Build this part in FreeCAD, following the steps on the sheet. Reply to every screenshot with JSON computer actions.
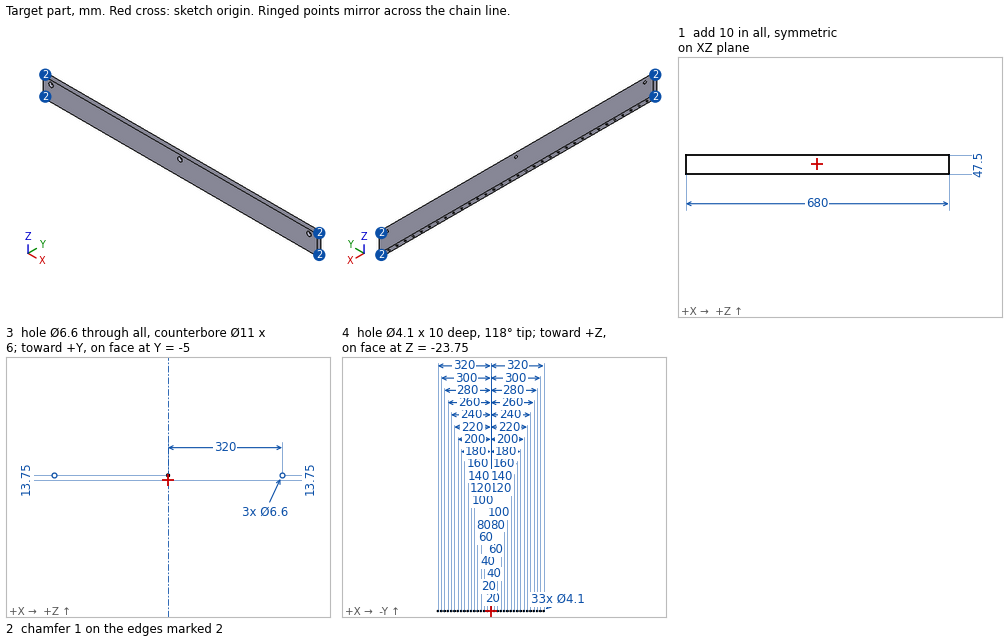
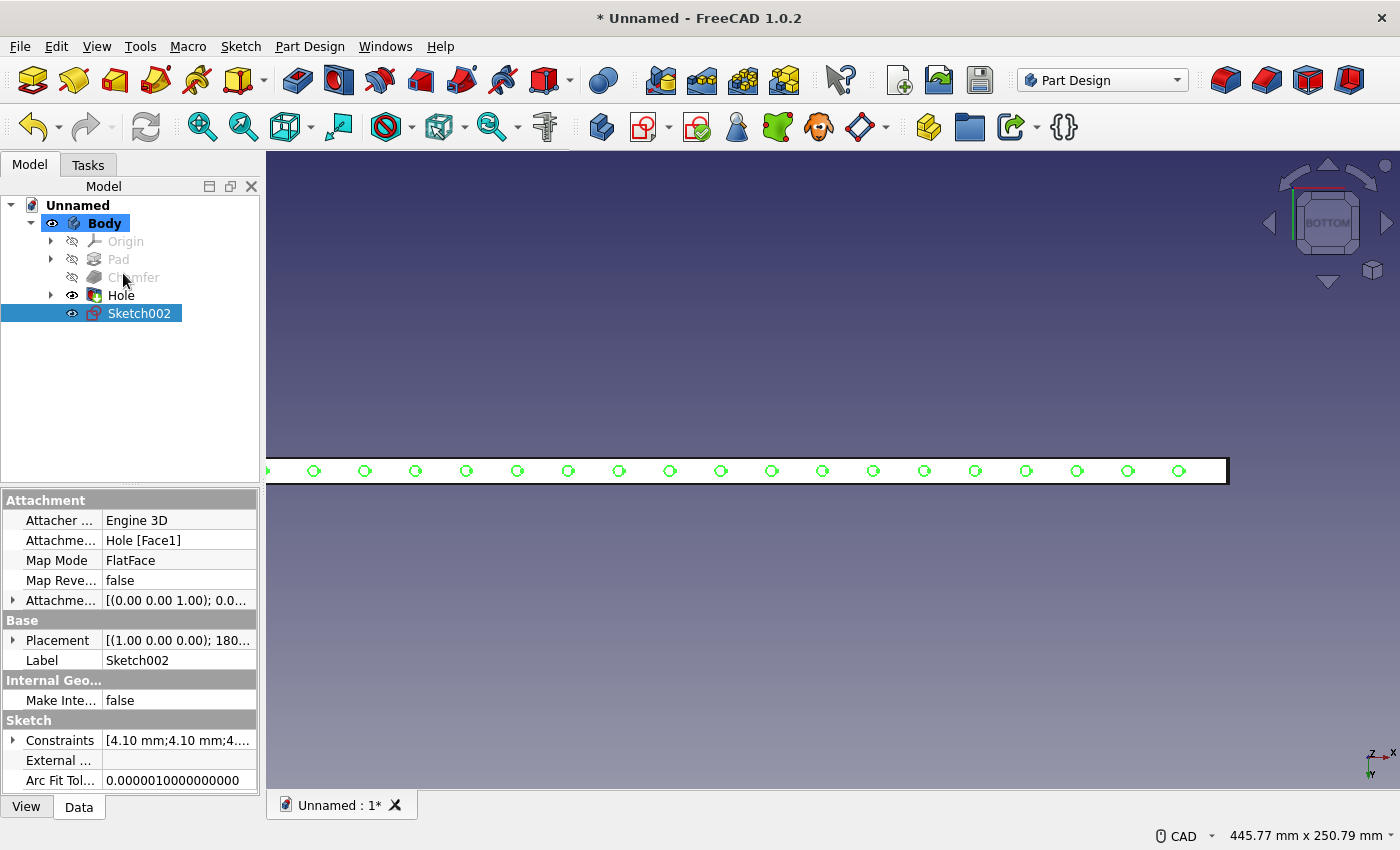
{"action": "left_click", "coordinate": [339, 80]}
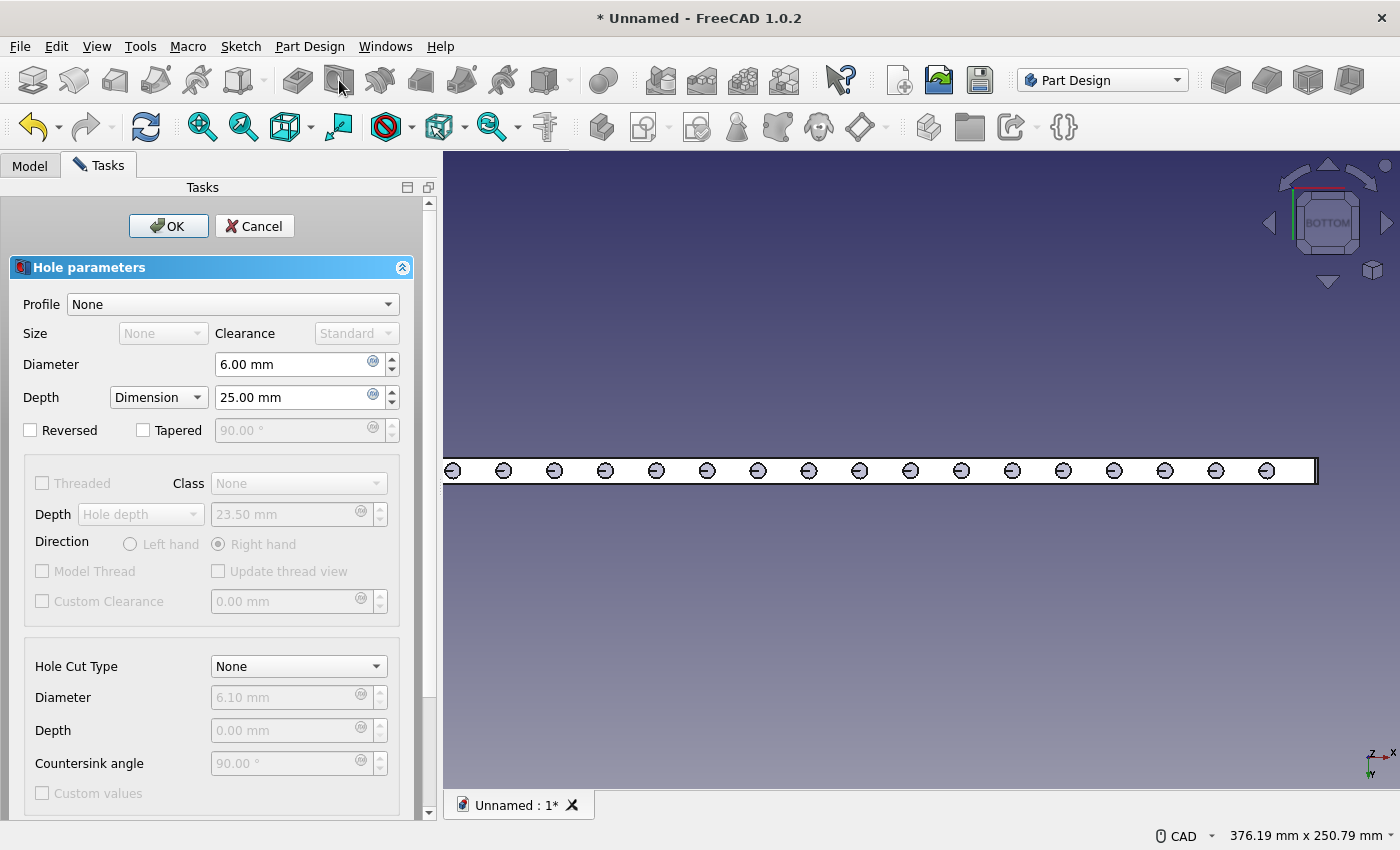
{"action": "triple_click", "coordinate": [300, 364]}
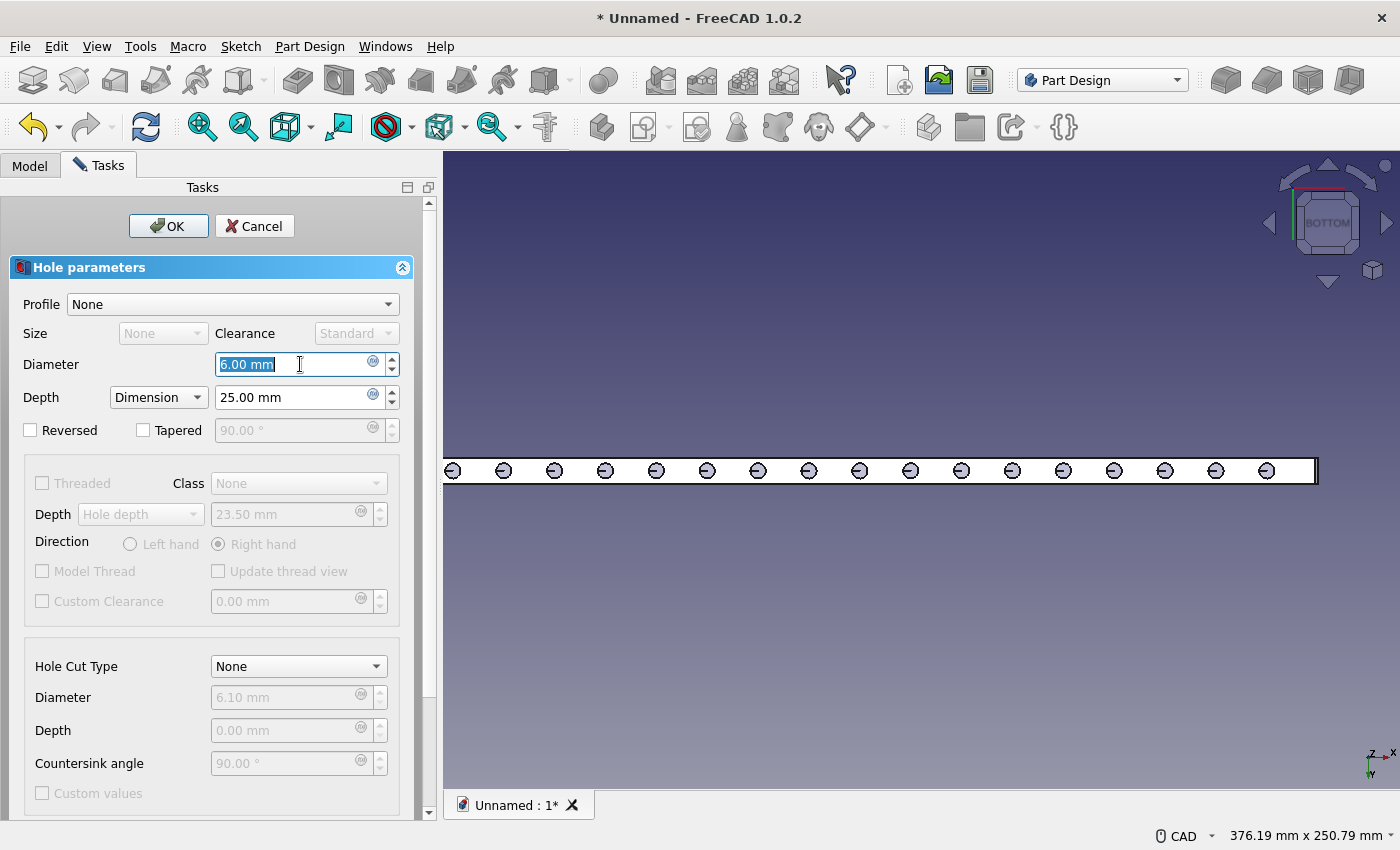
{"action": "type", "text": "4.1"}
{"action": "key", "text": "Tab"}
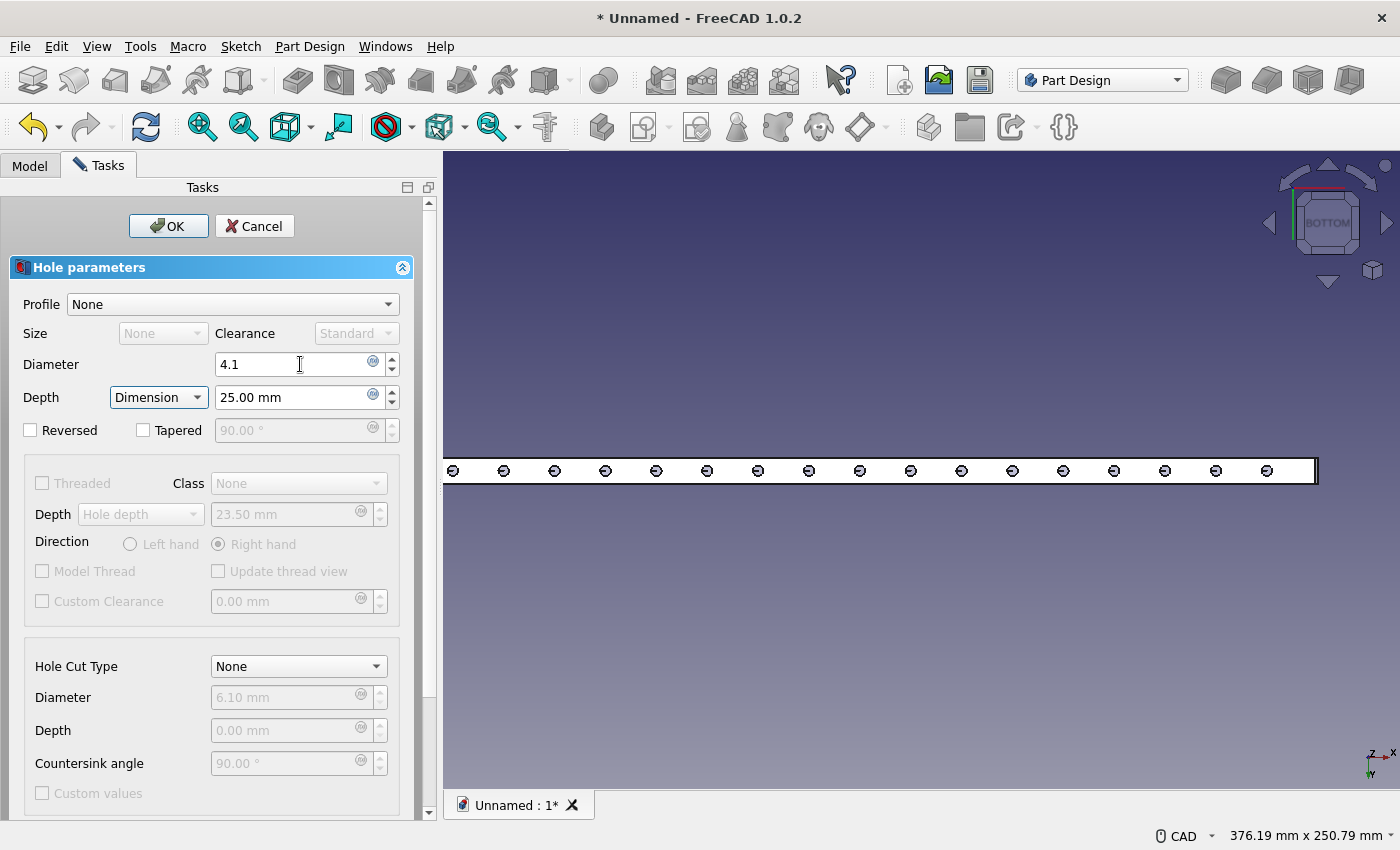
{"action": "triple_click", "coordinate": [300, 398]}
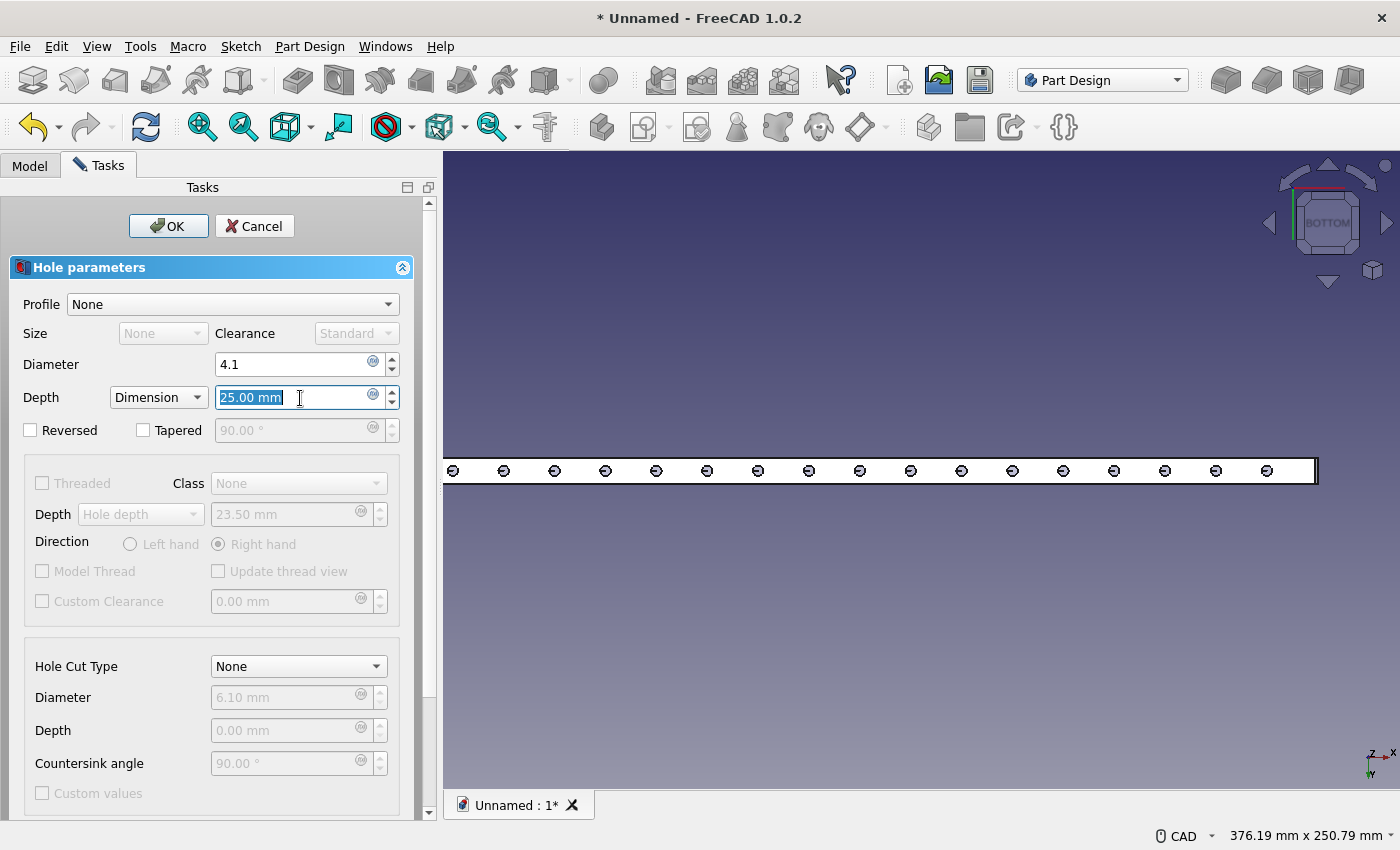
{"action": "type", "text": "10"}
{"action": "key", "text": "Tab"}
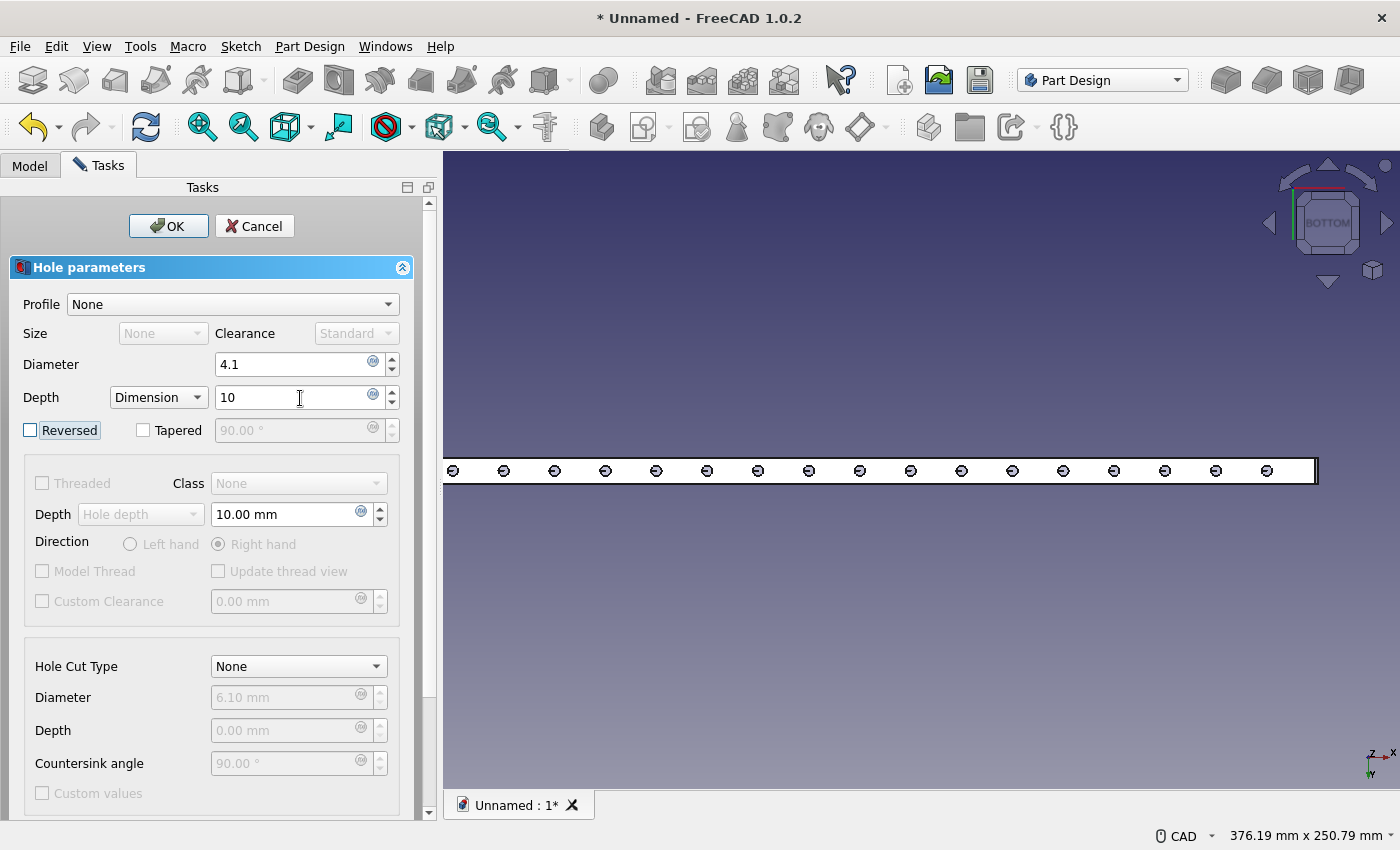
{"action": "left_click", "coordinate": [169, 226]}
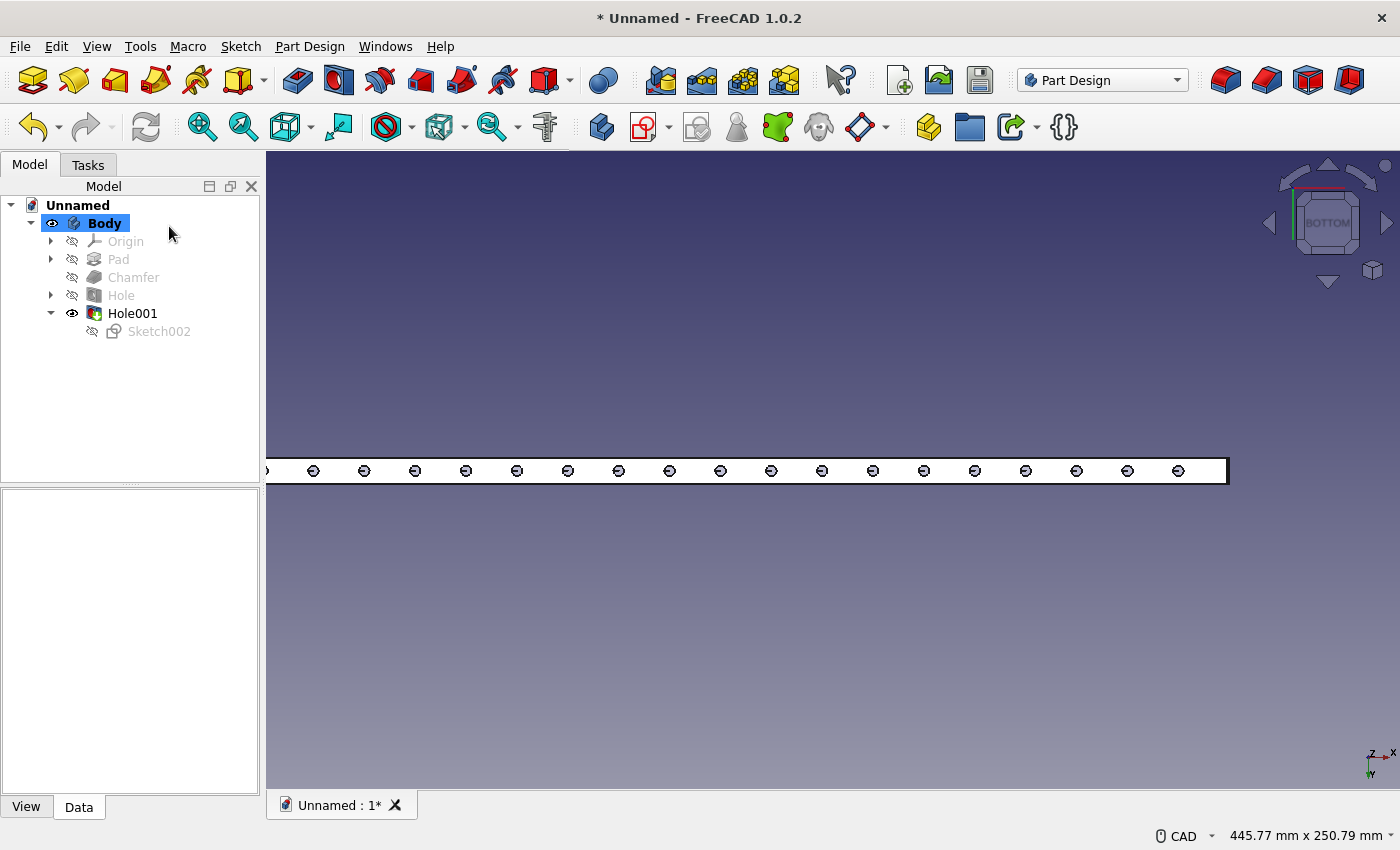
{"action": "key", "text": "0"}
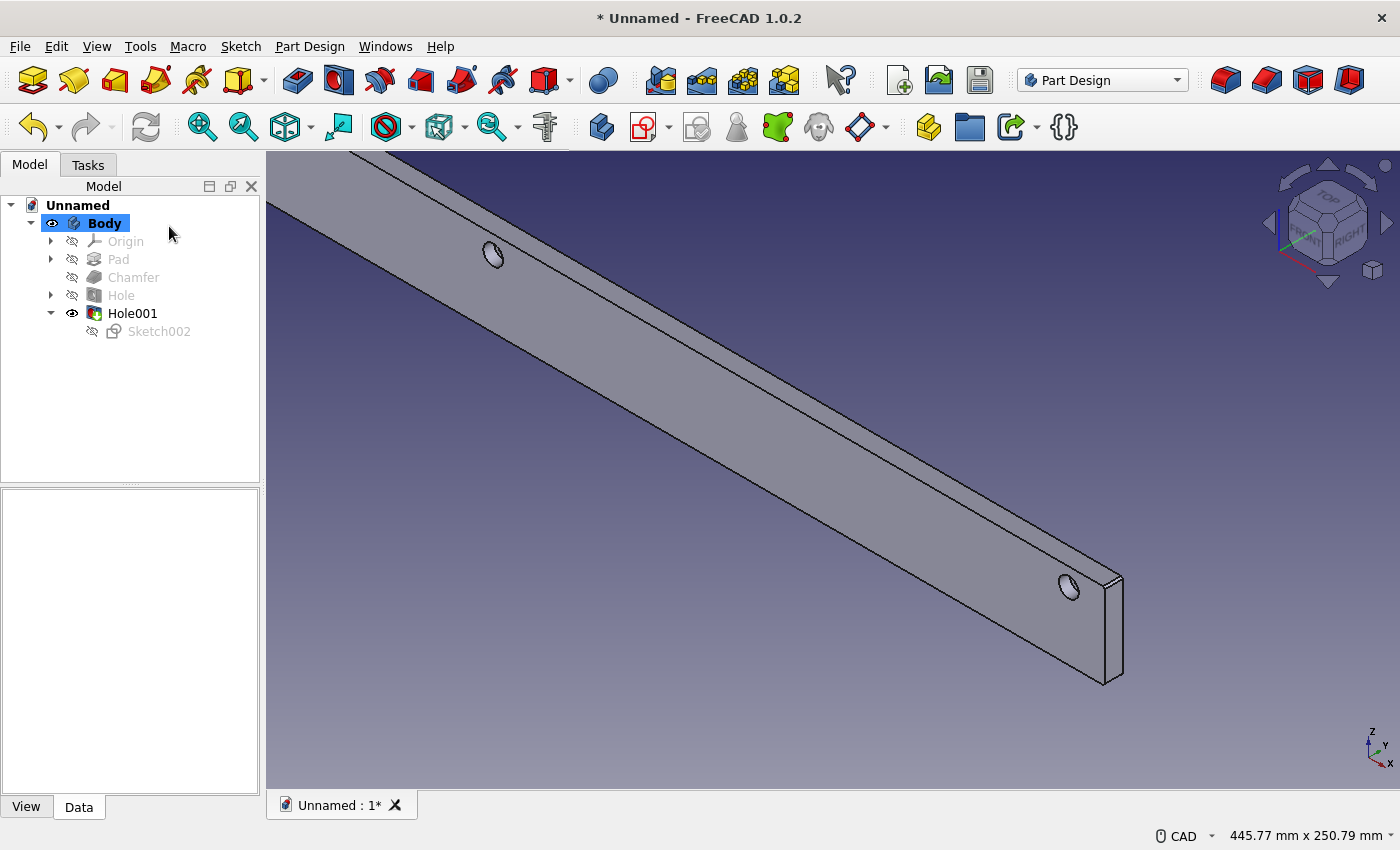
{"action": "left_click", "coordinate": [203, 128]}